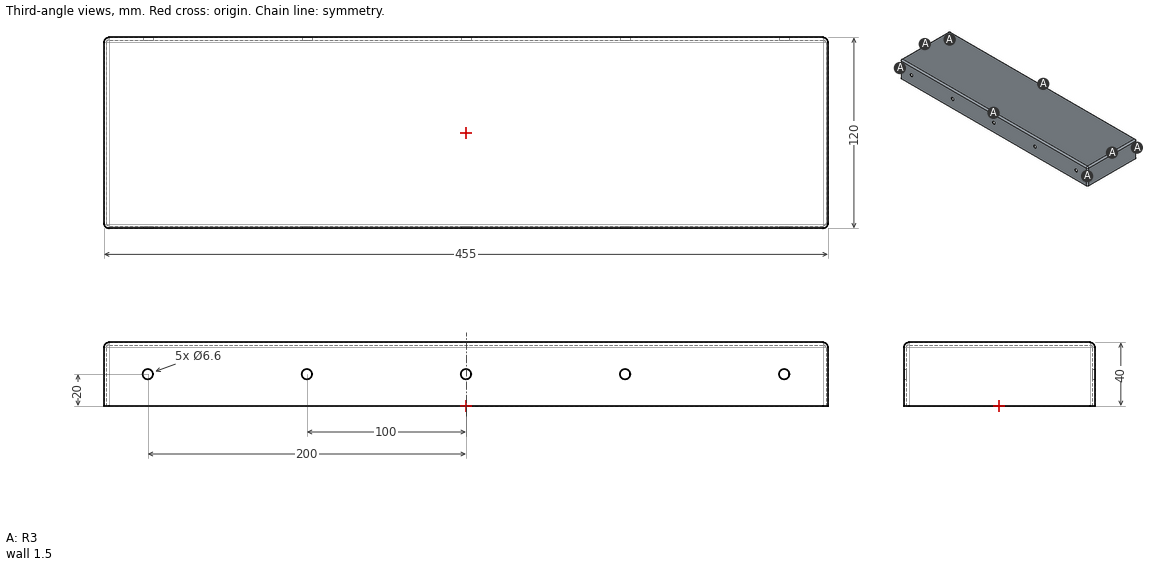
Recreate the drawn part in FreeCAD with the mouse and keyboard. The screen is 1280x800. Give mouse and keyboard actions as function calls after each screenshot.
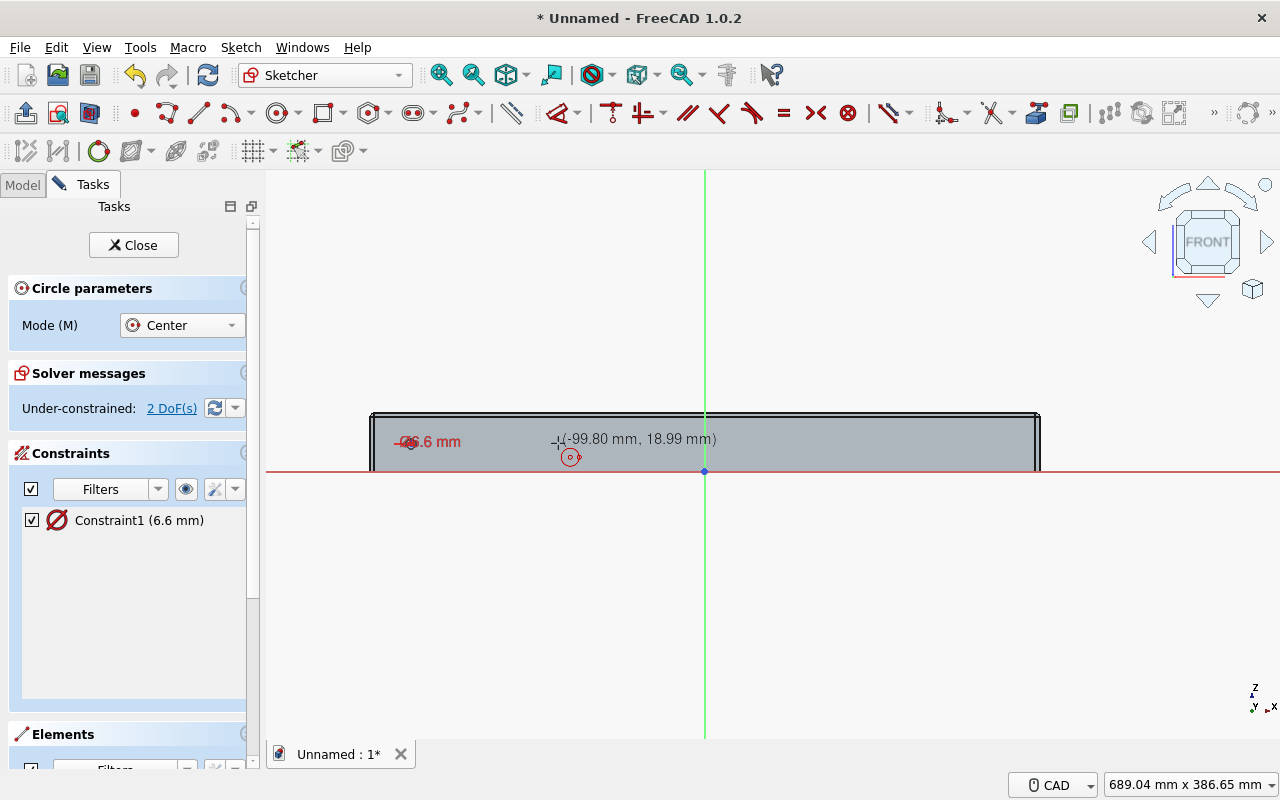
click(558, 443)
move(561, 439)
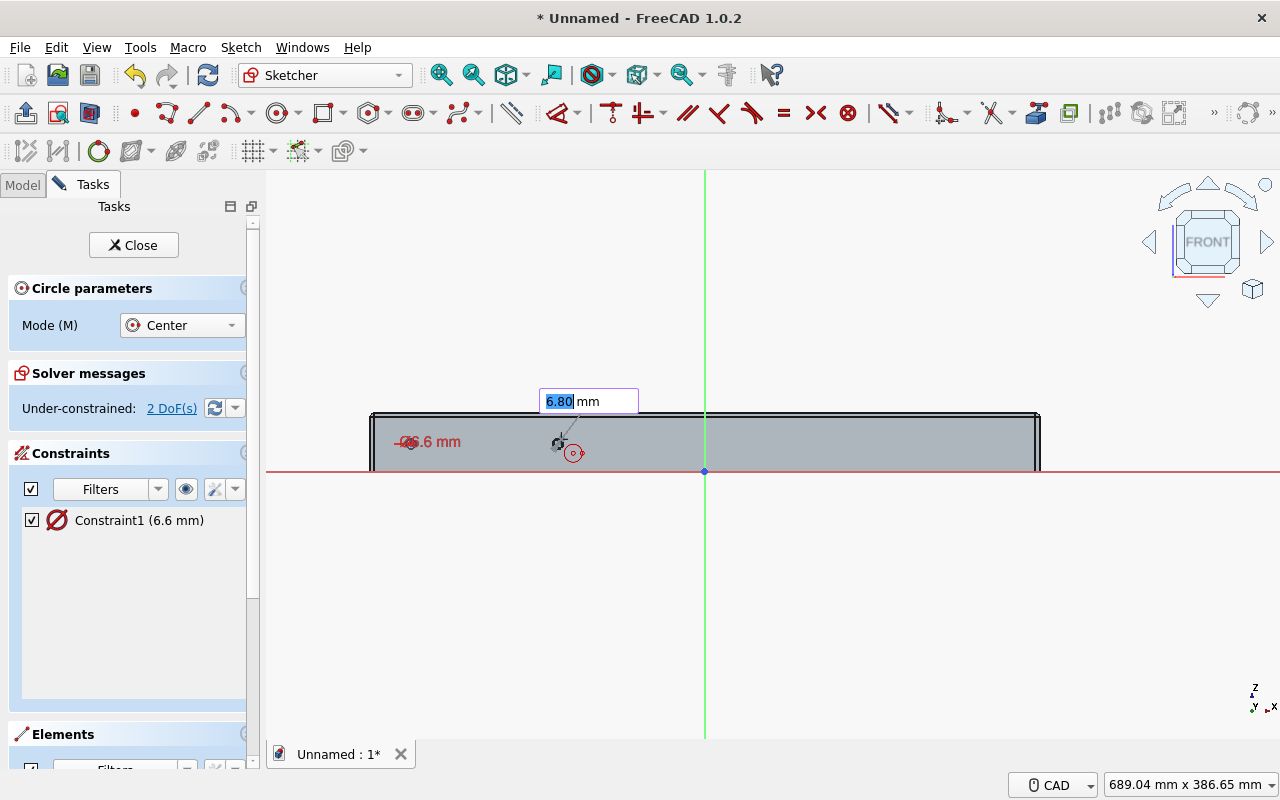
text(6.6)
key(Return)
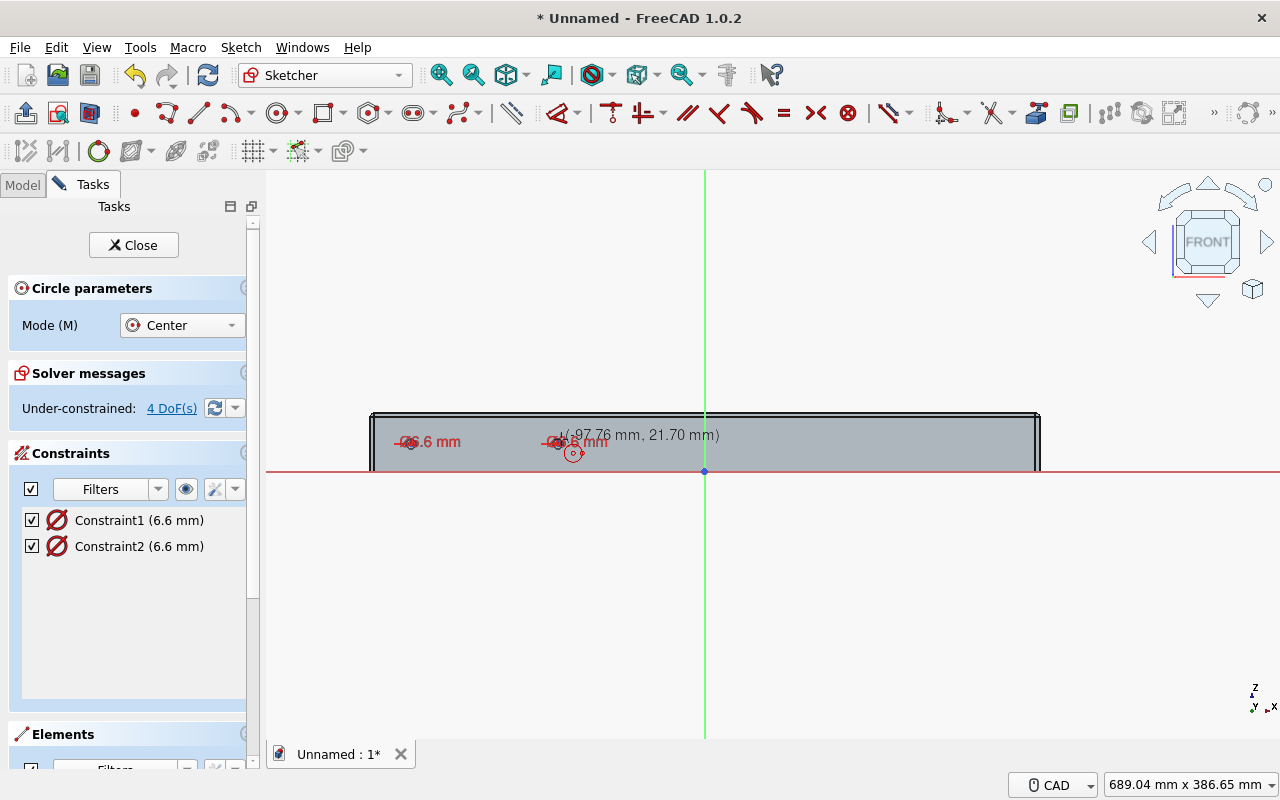
scroll(852, 443, up, 8)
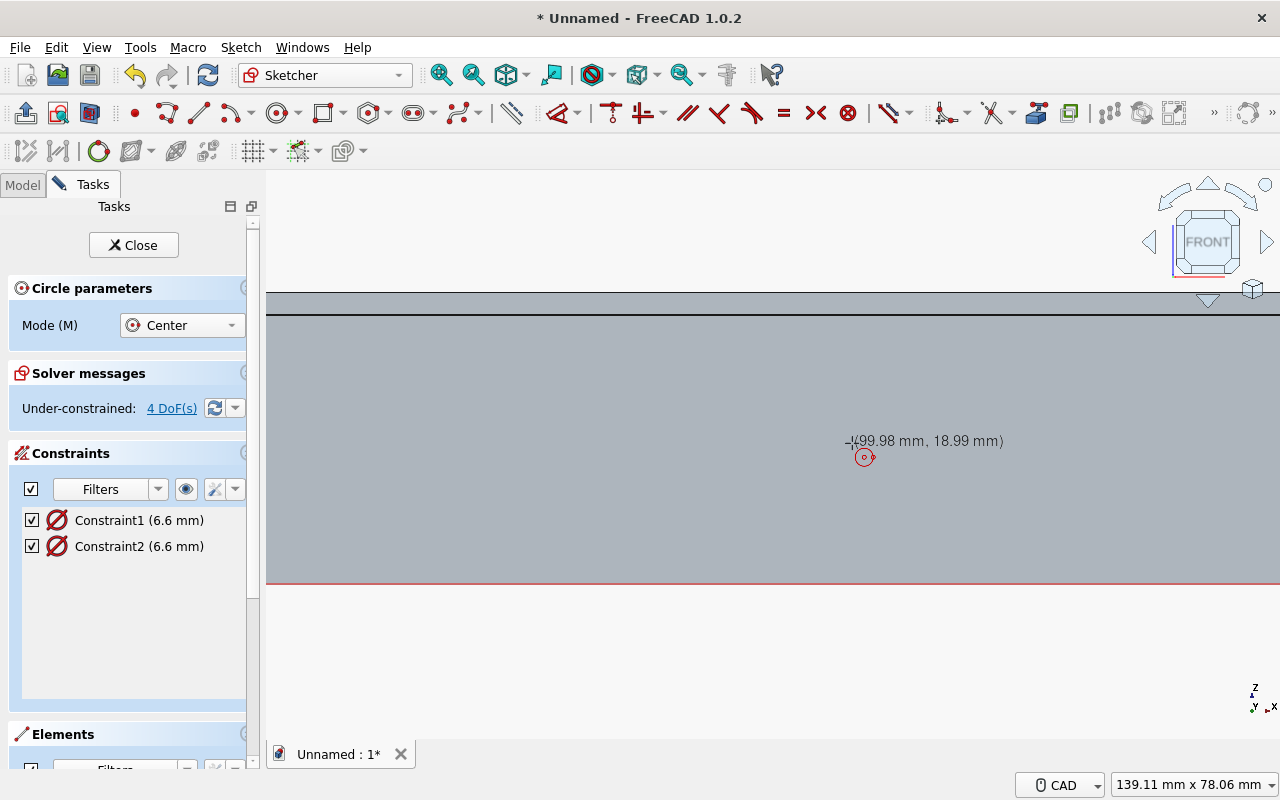
scroll(852, 443, down, 8)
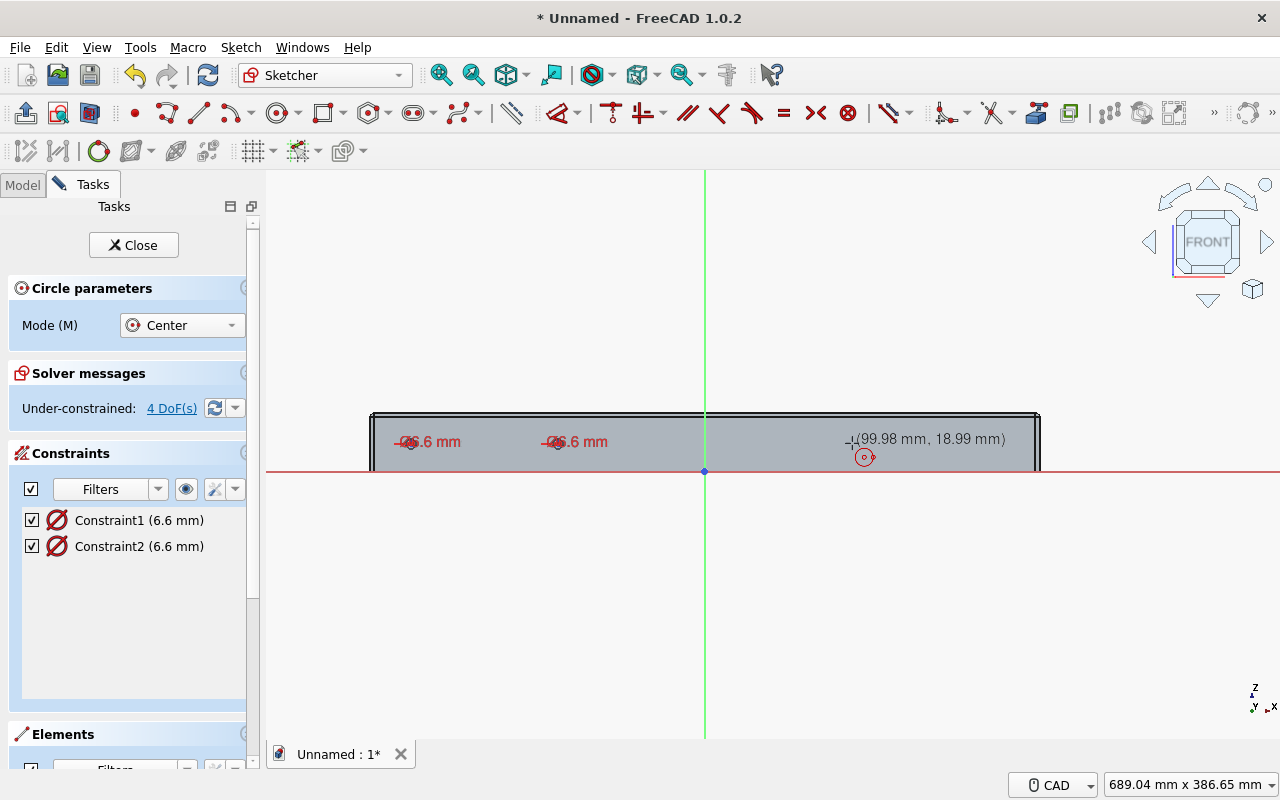
click(852, 443)
move(855, 439)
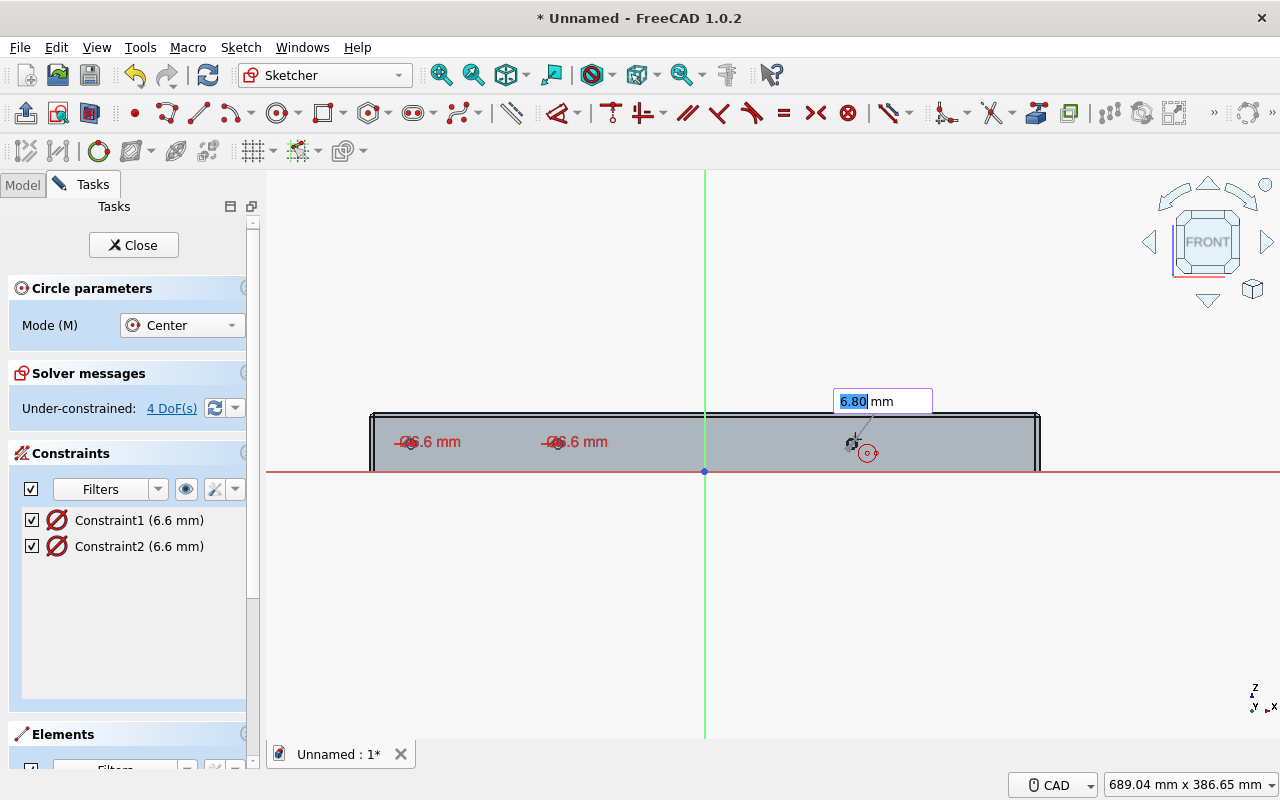
text(6.6)
key(Return)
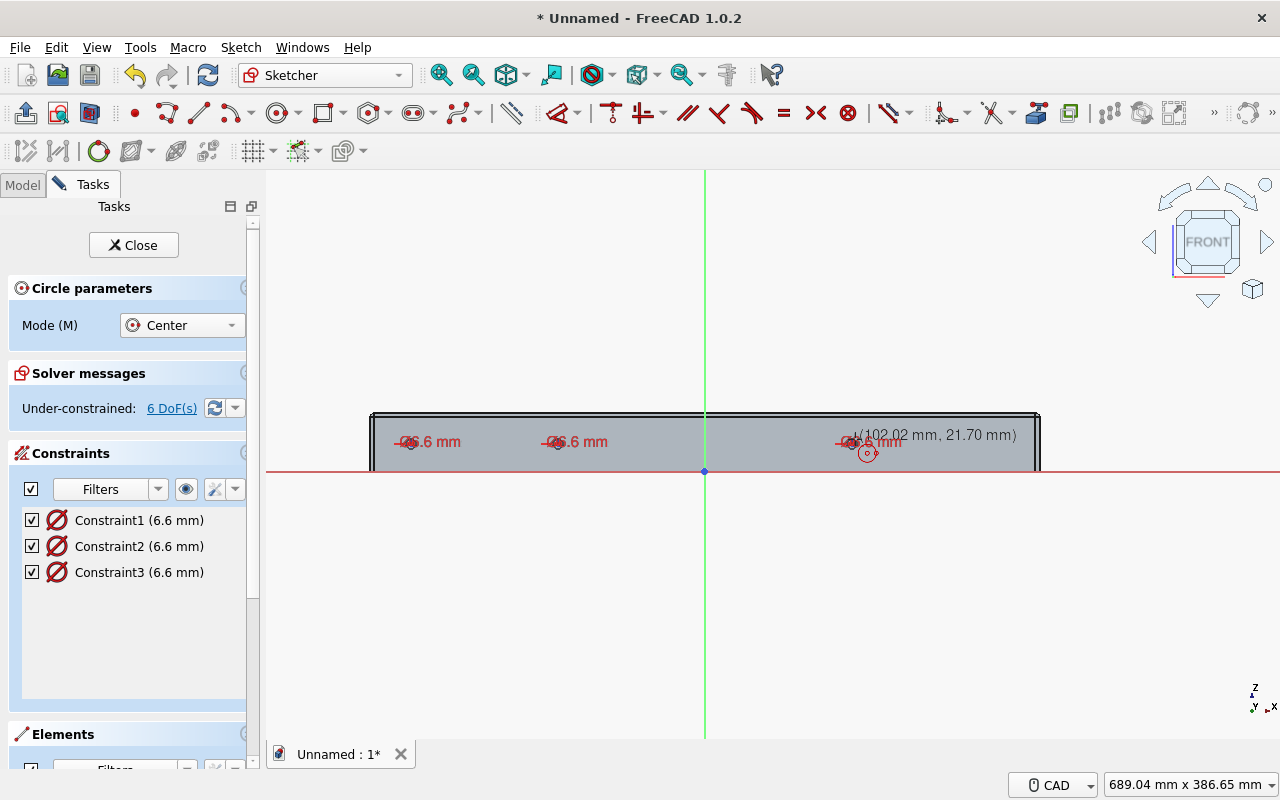
scroll(999, 443, up, 8)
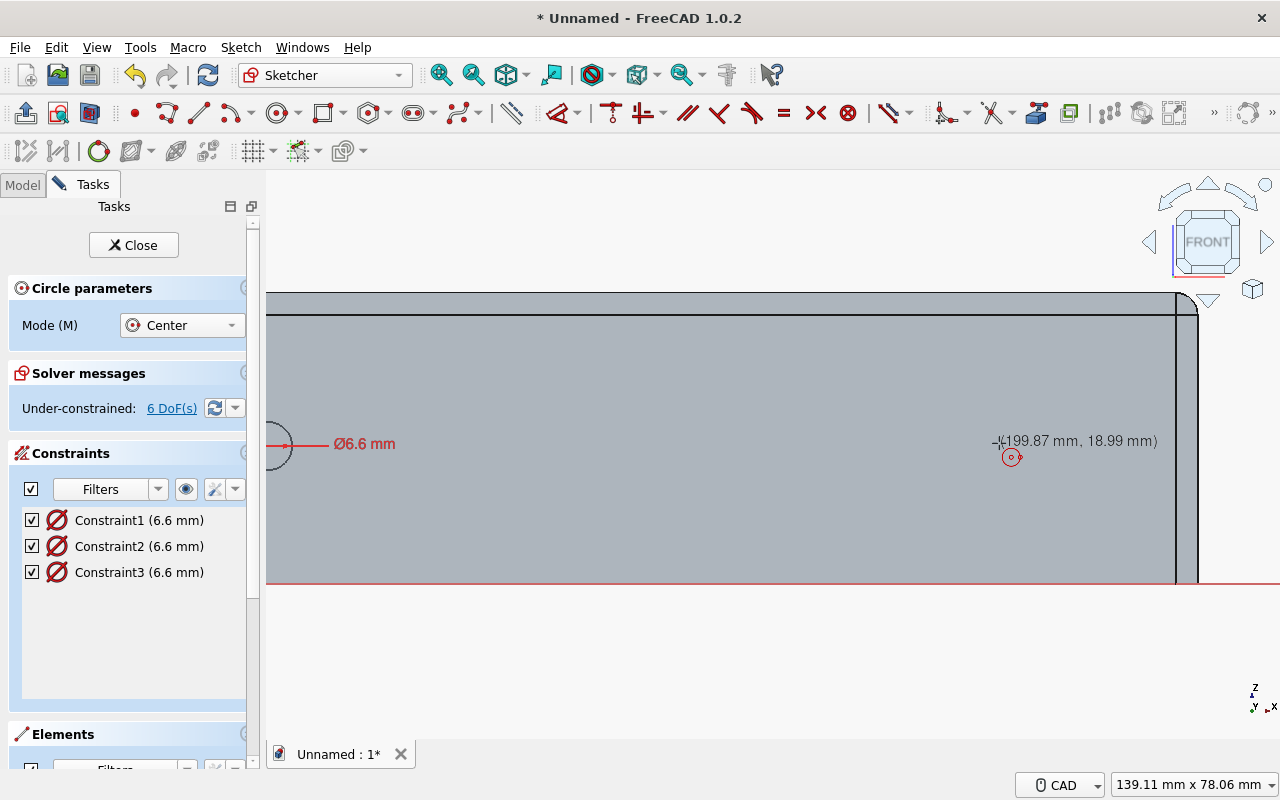
scroll(999, 443, down, 8)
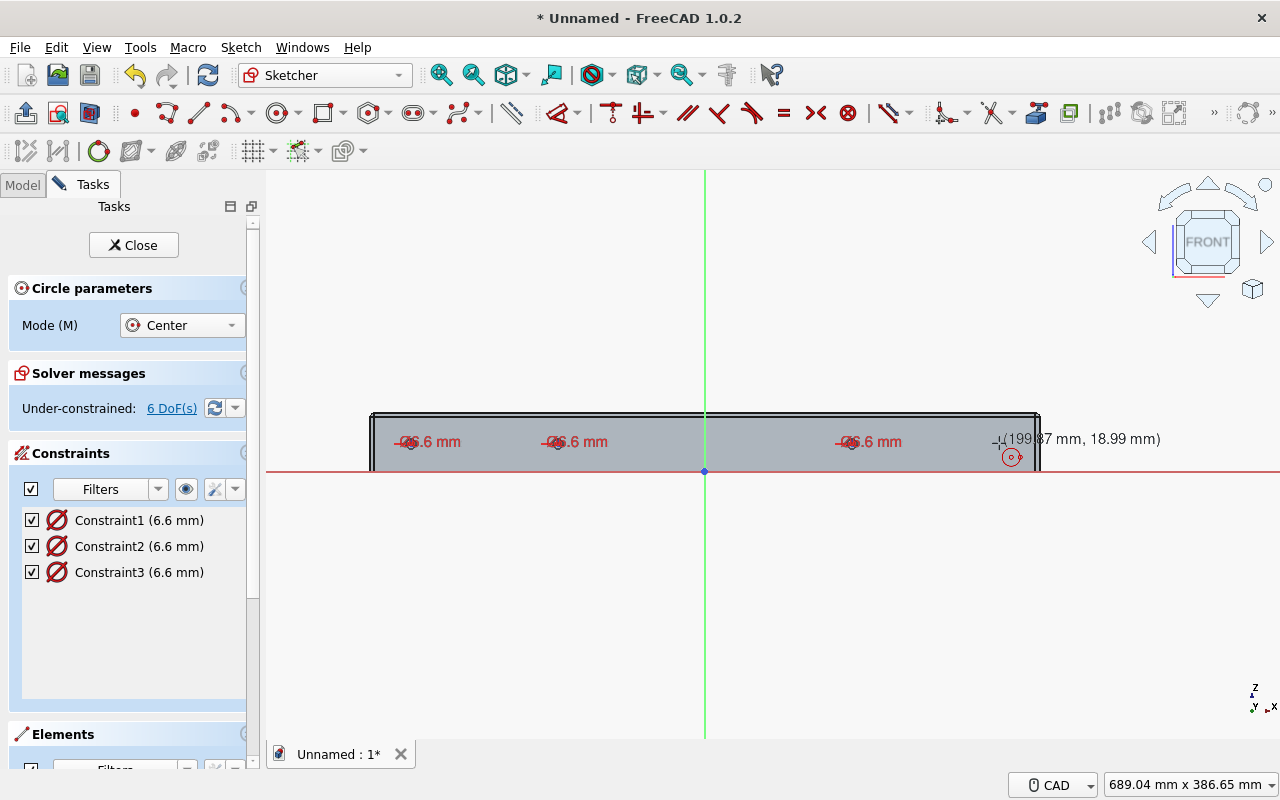
click(999, 443)
move(1003, 439)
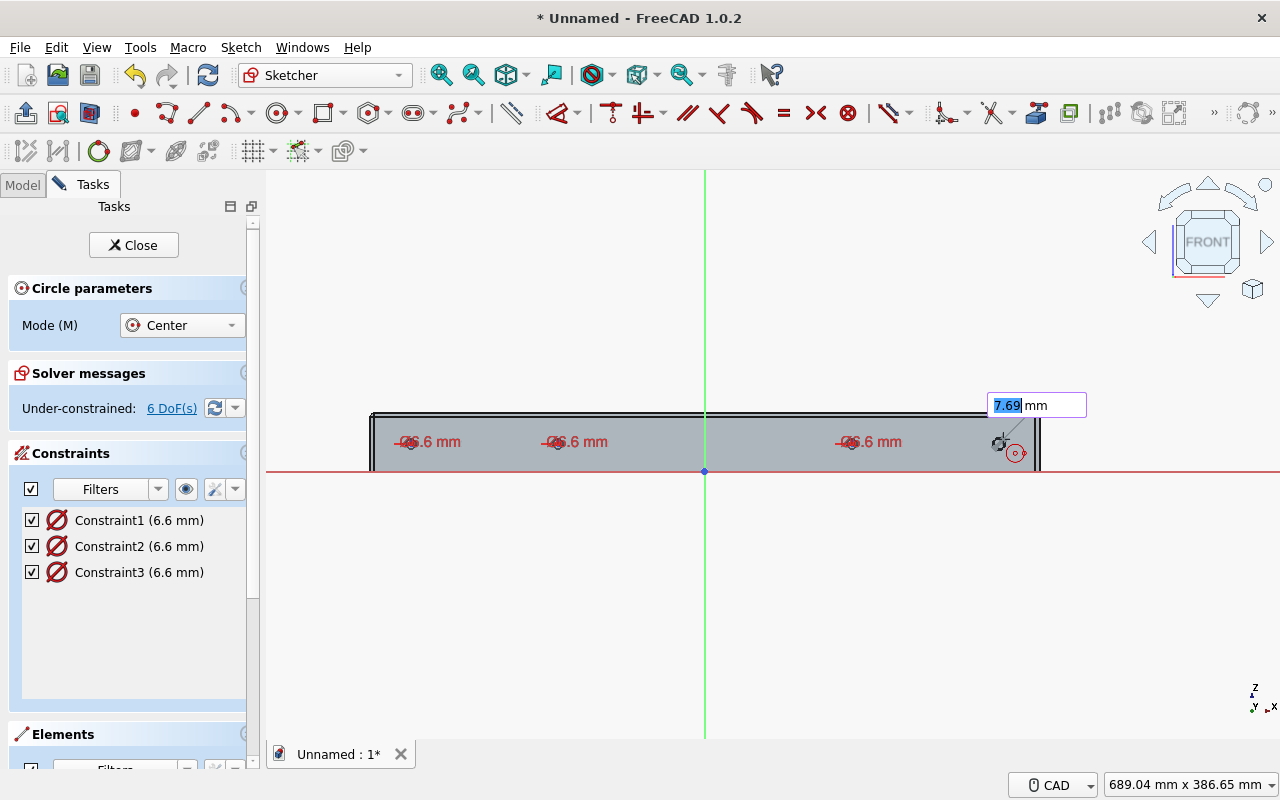
text(6.6)
key(Return)